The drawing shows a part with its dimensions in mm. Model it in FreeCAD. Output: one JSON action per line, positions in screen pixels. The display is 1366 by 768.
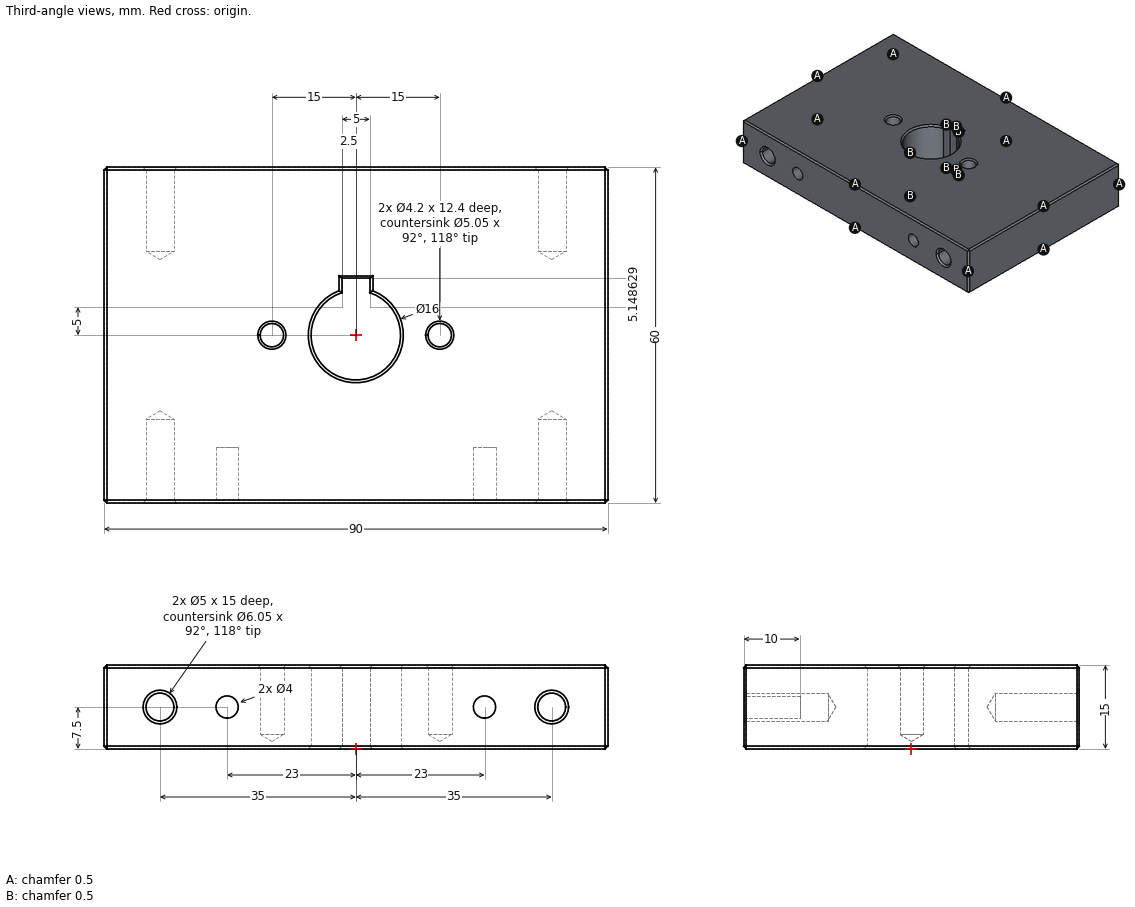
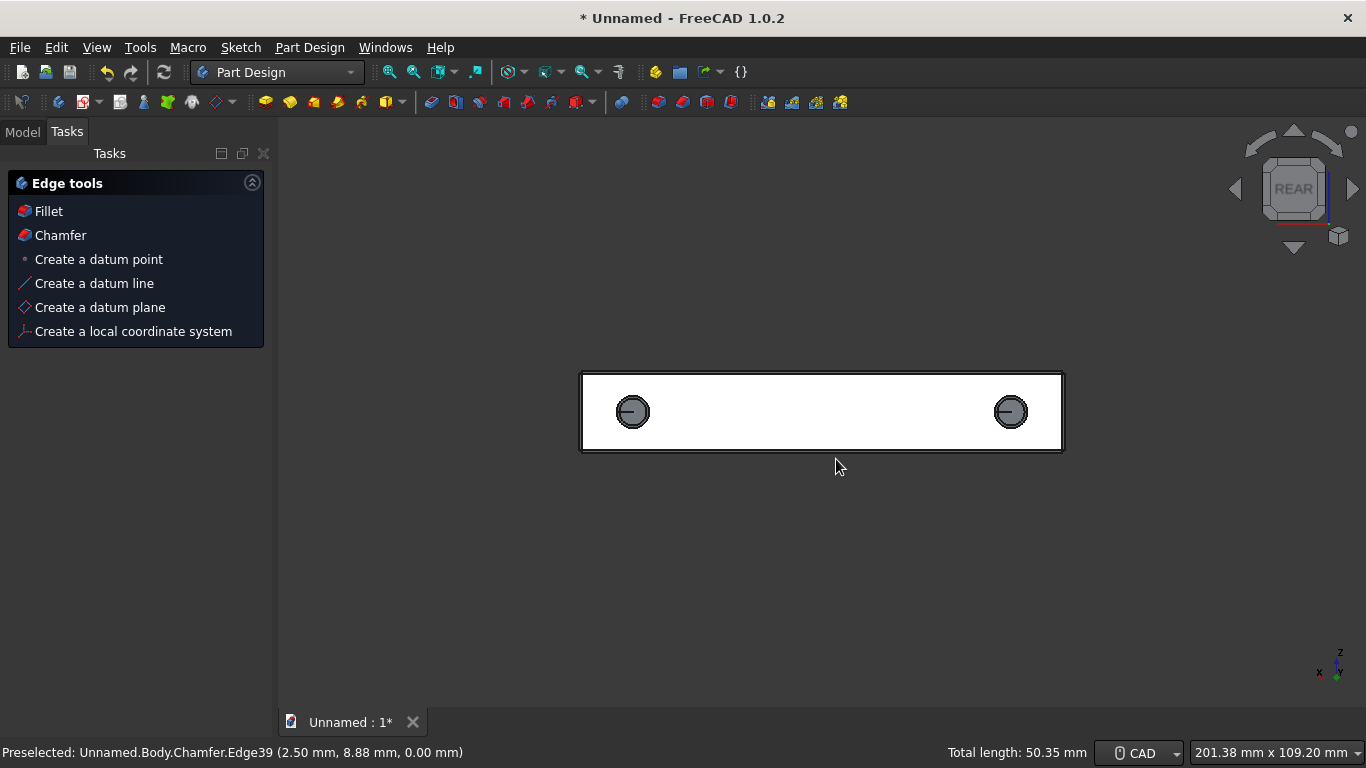
{"action": "key", "text": "v f"}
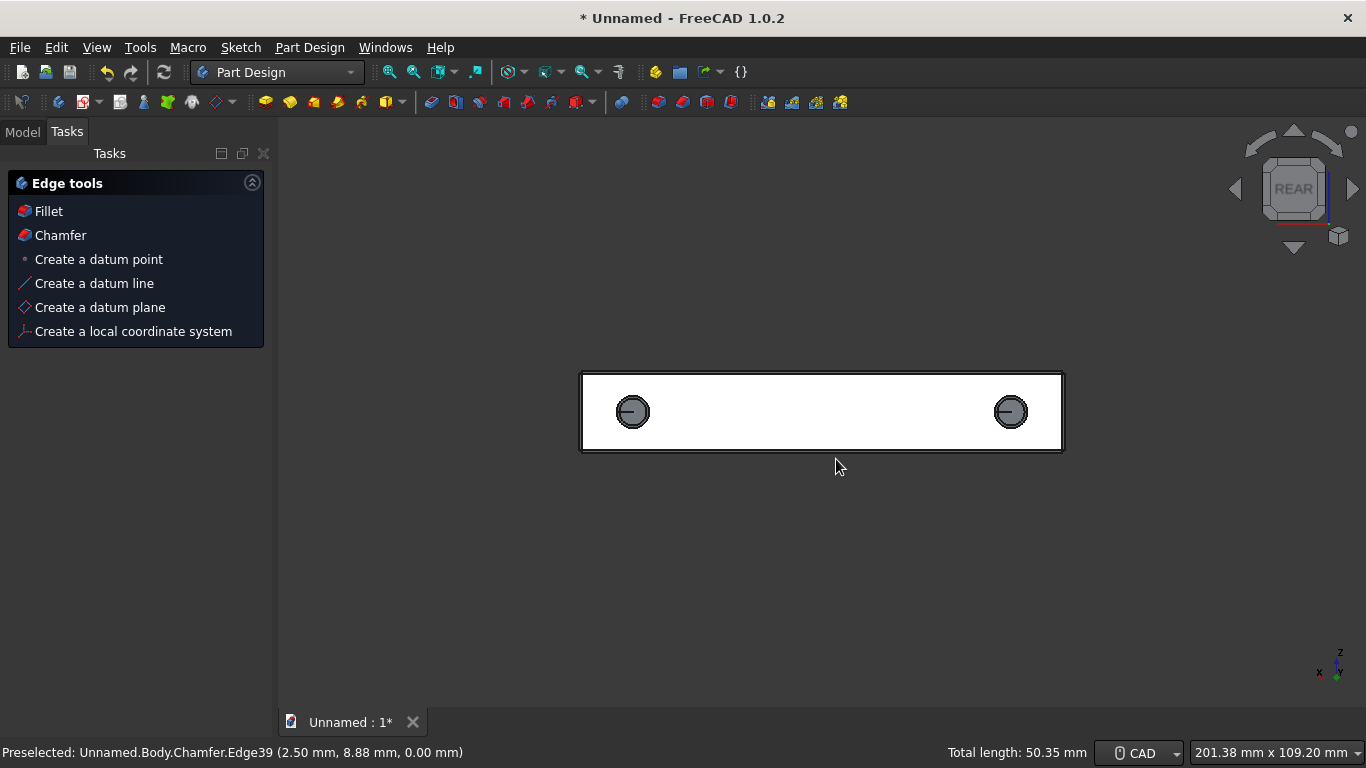
{"action": "key", "text": "6"}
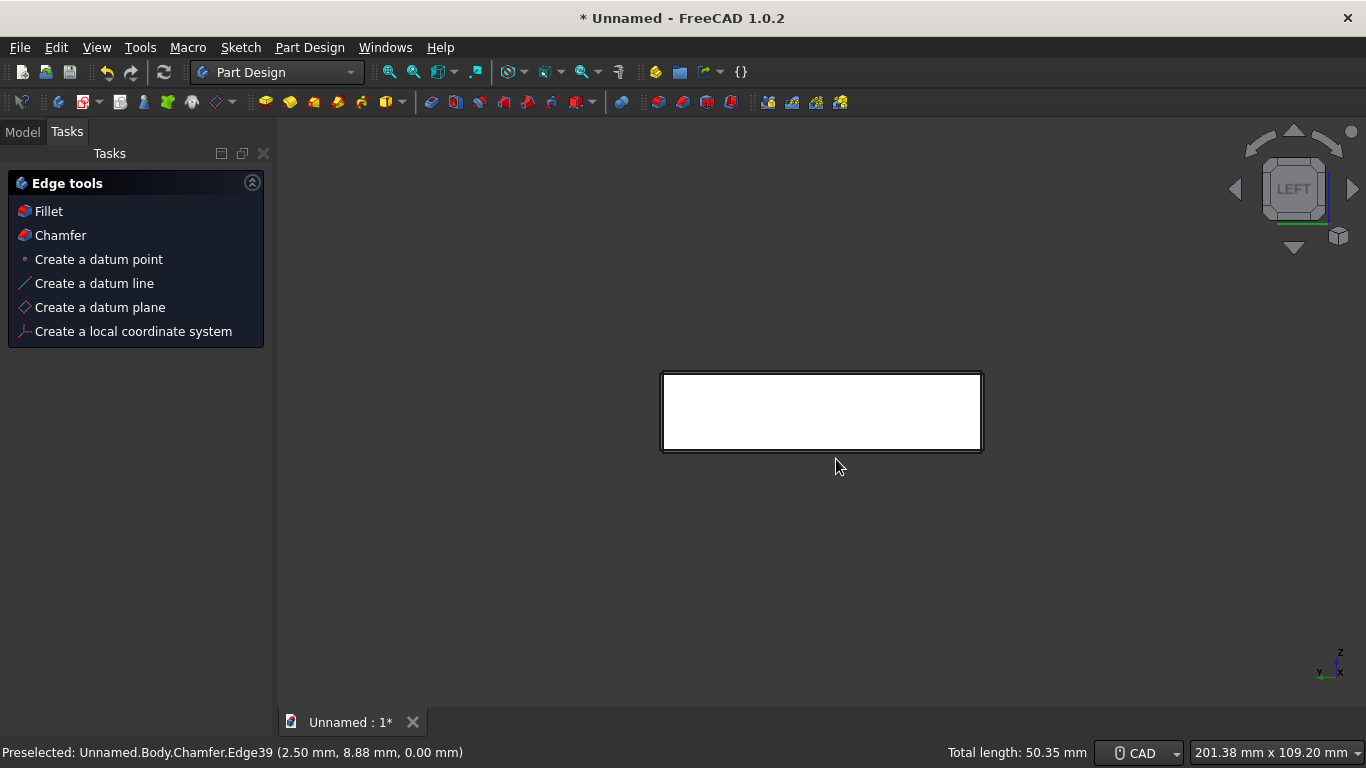
{"action": "key", "text": "v f"}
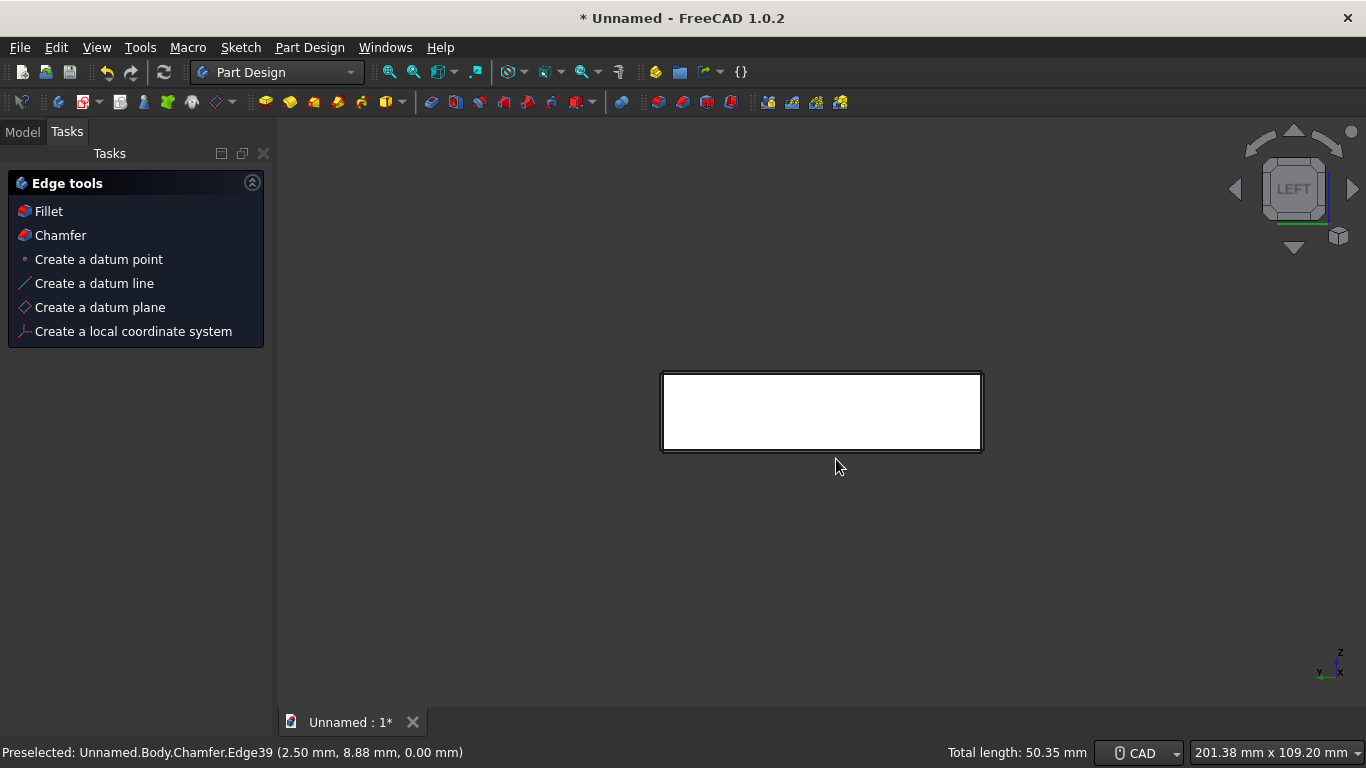
{"action": "key", "text": "v 3"}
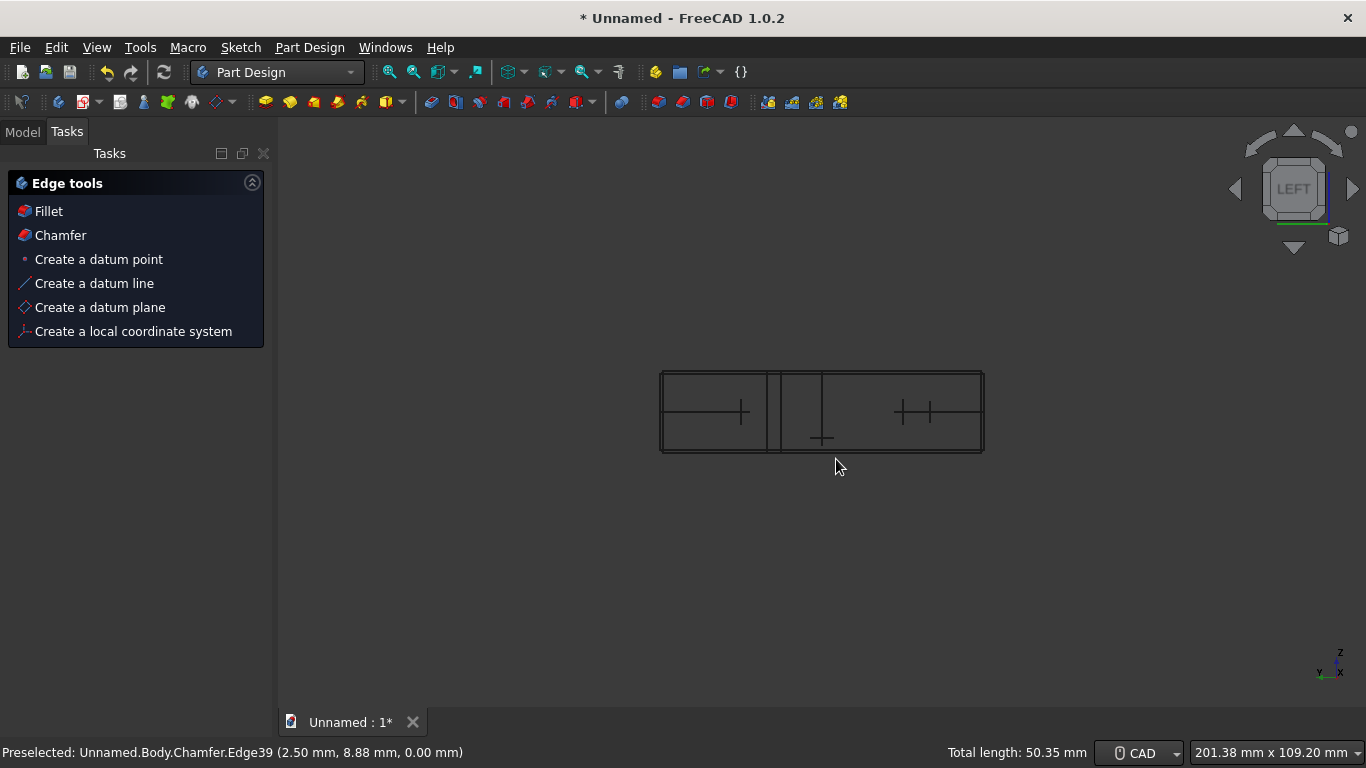
{"action": "key", "text": "0"}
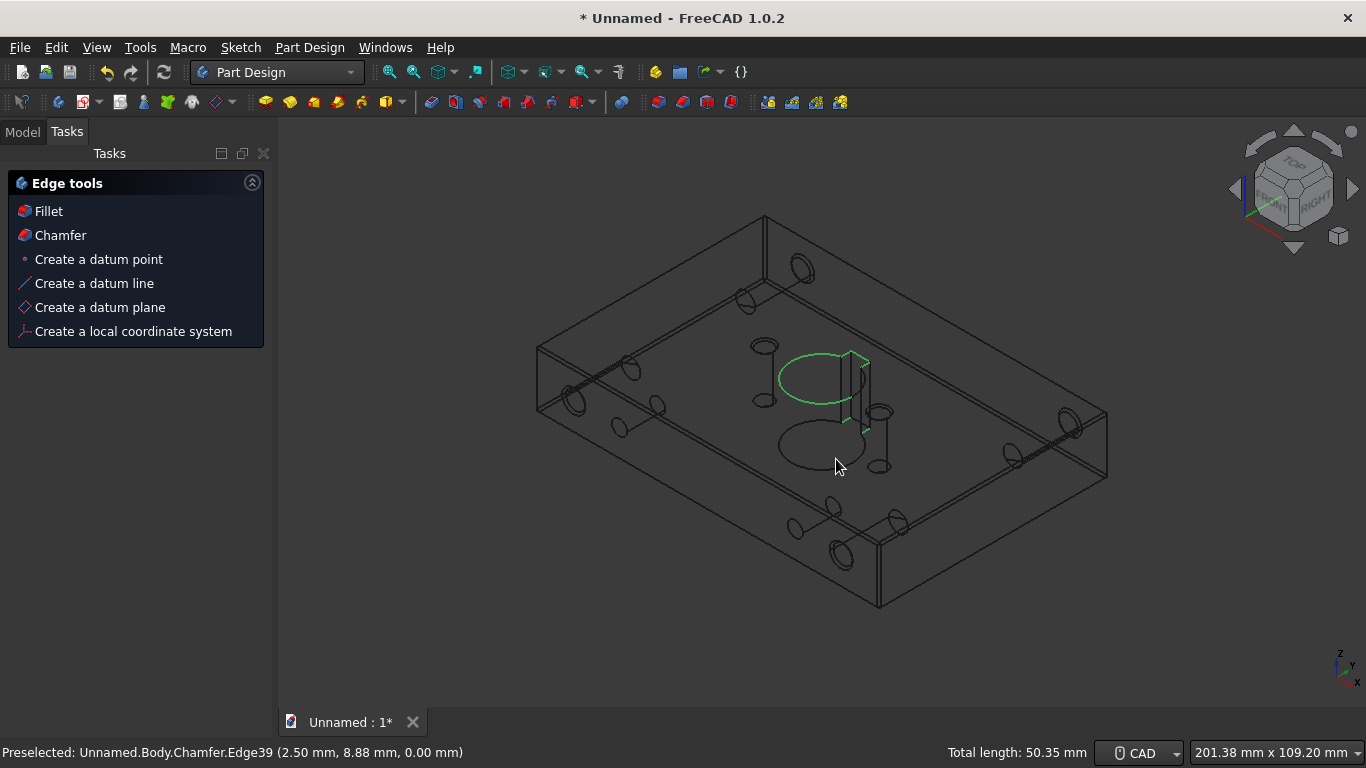
{"action": "left_click", "coordinate": [779, 448], "text": "ctrl"}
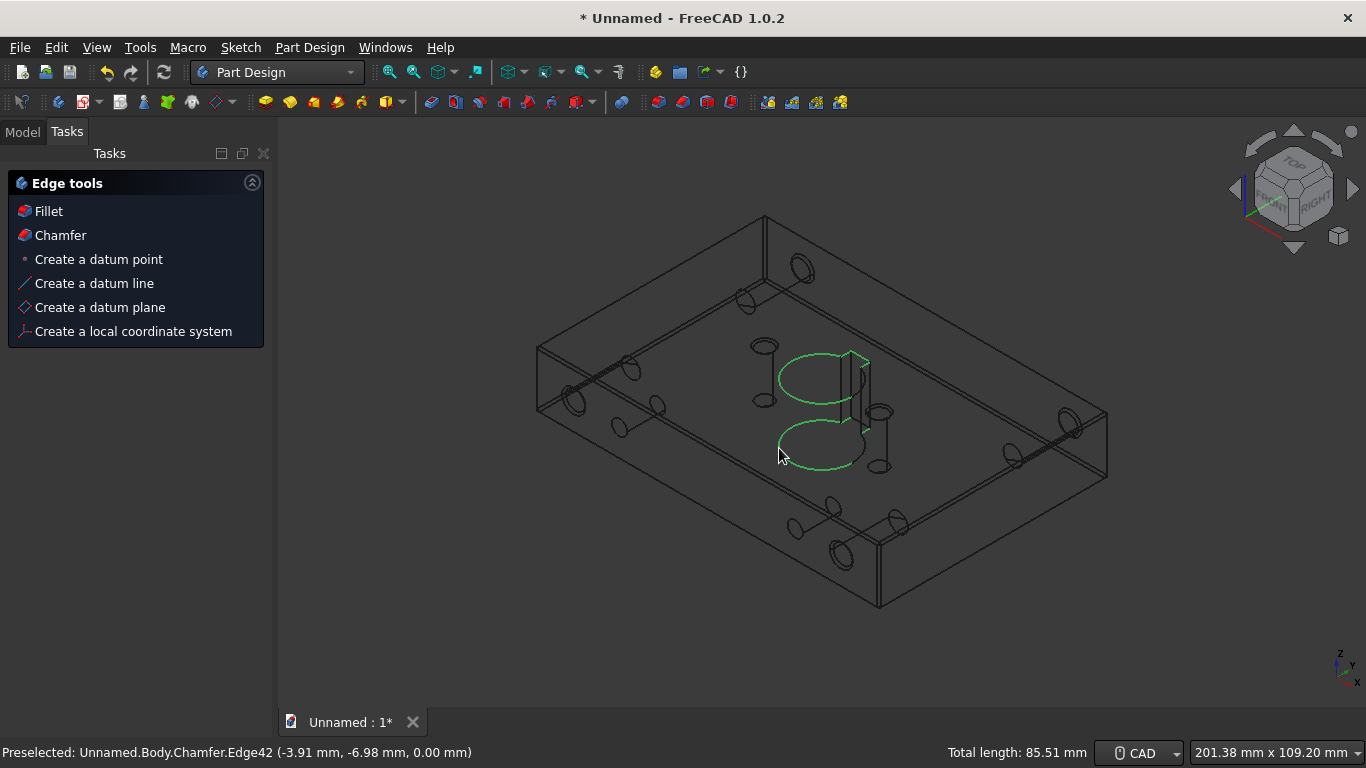
{"action": "left_click", "coordinate": [854, 418], "text": "ctrl"}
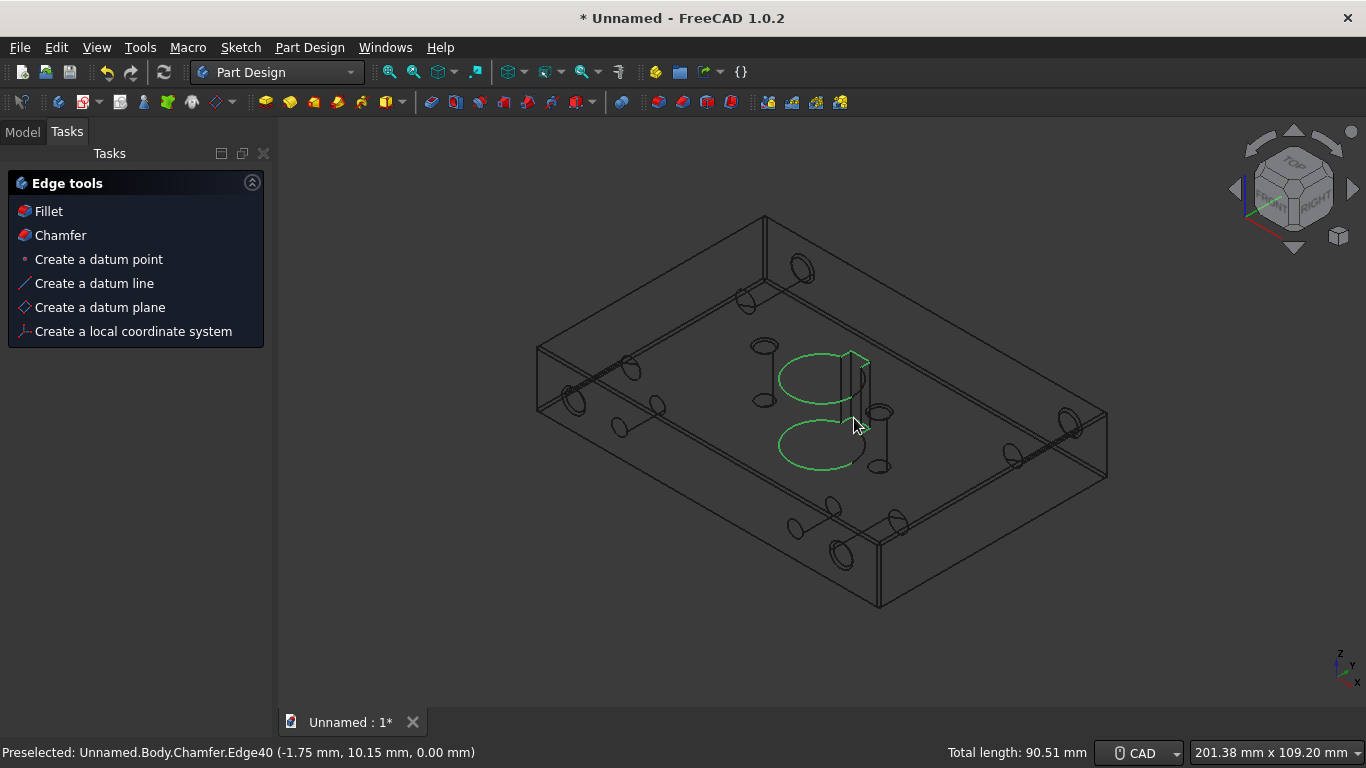
{"action": "key", "text": "v 1"}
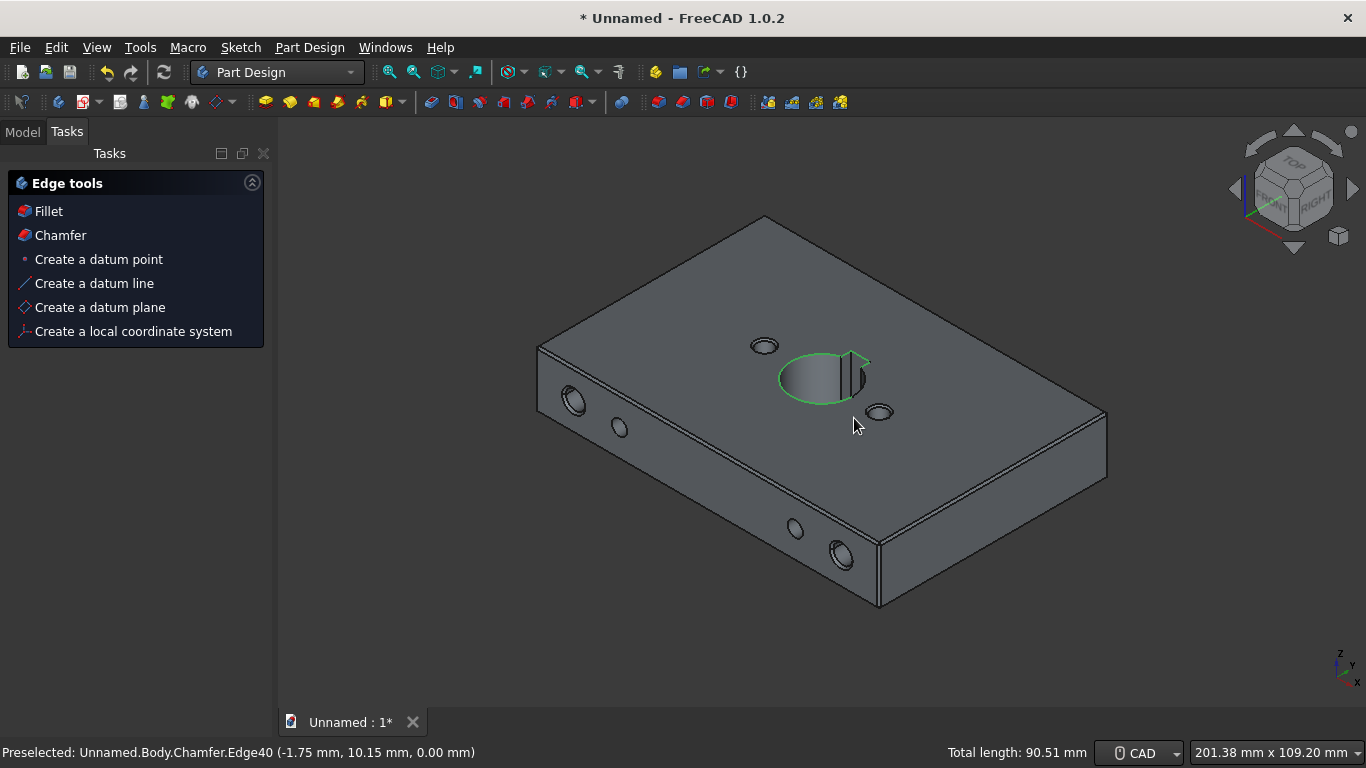
{"action": "left_click", "coordinate": [684, 102]}